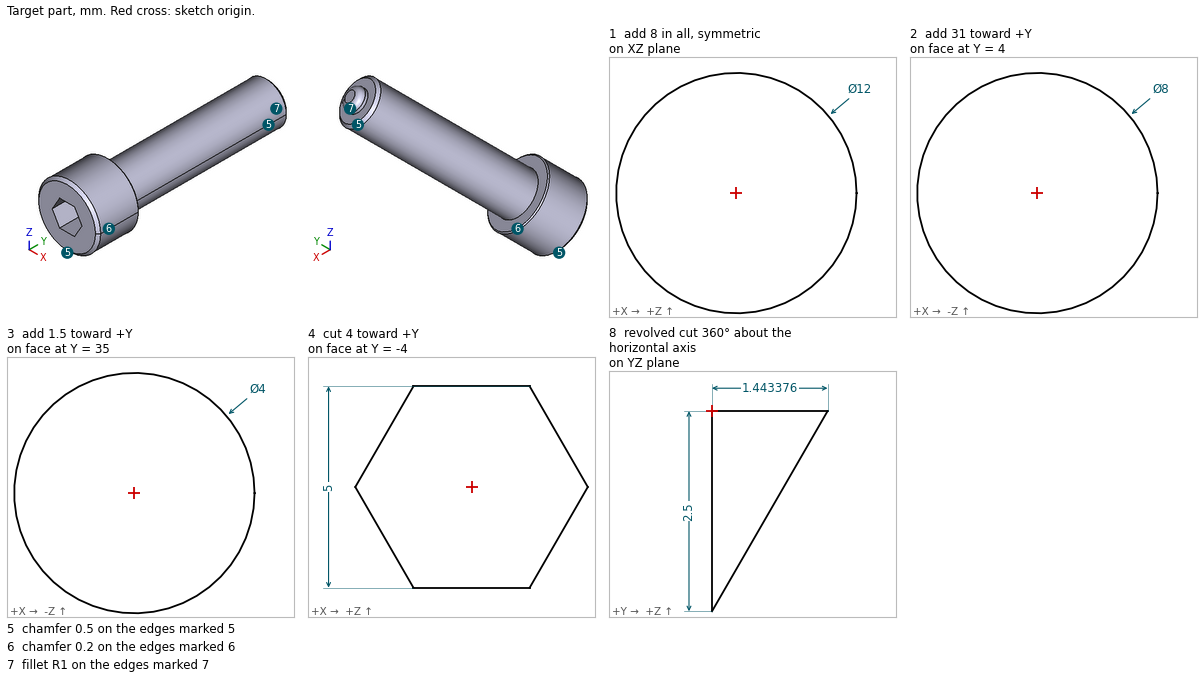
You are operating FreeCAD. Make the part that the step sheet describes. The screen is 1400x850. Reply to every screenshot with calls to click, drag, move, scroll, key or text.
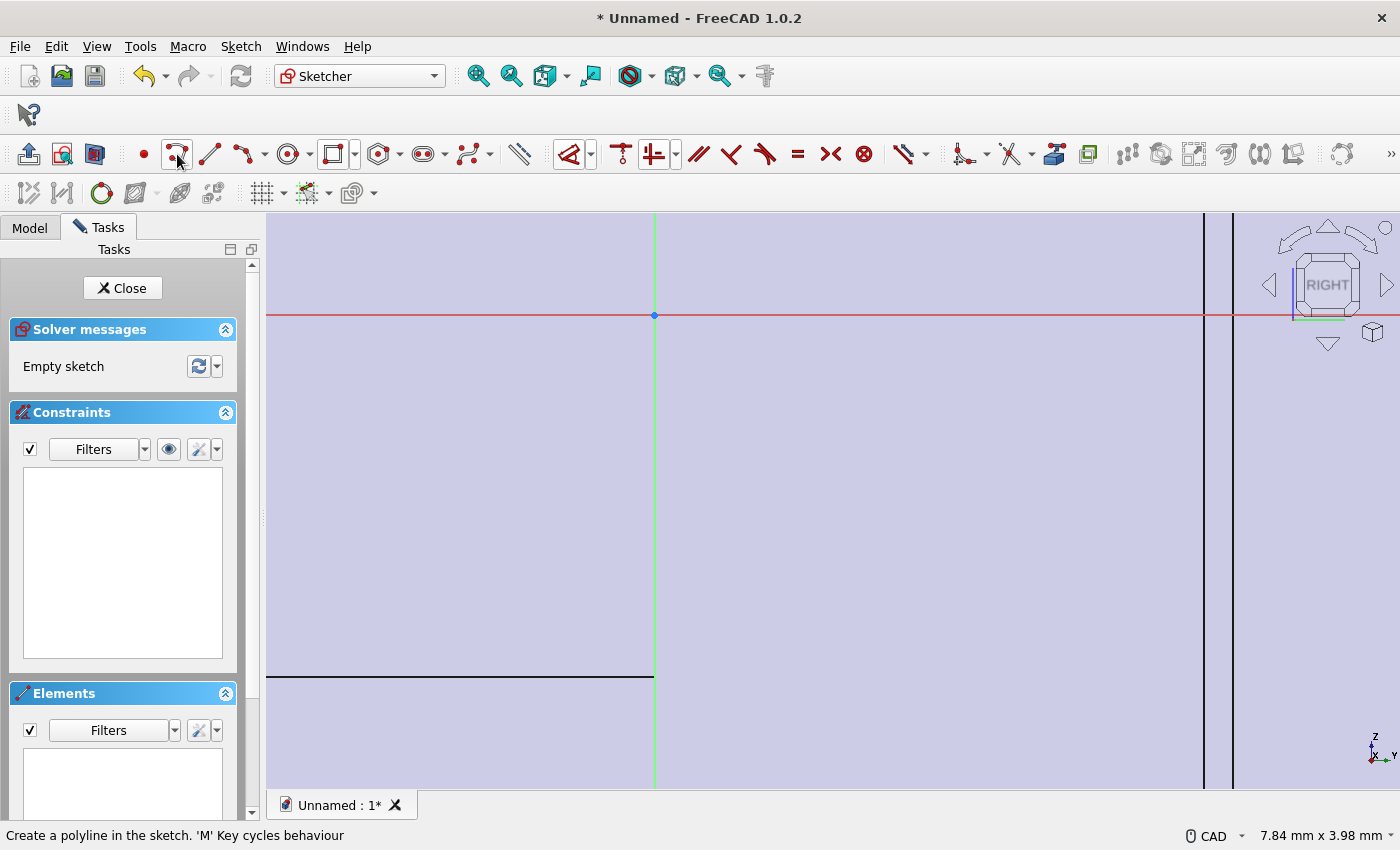
click(655, 315)
click(664, 677)
click(863, 324)
click(655, 315)
key(Escape)
key(Escape)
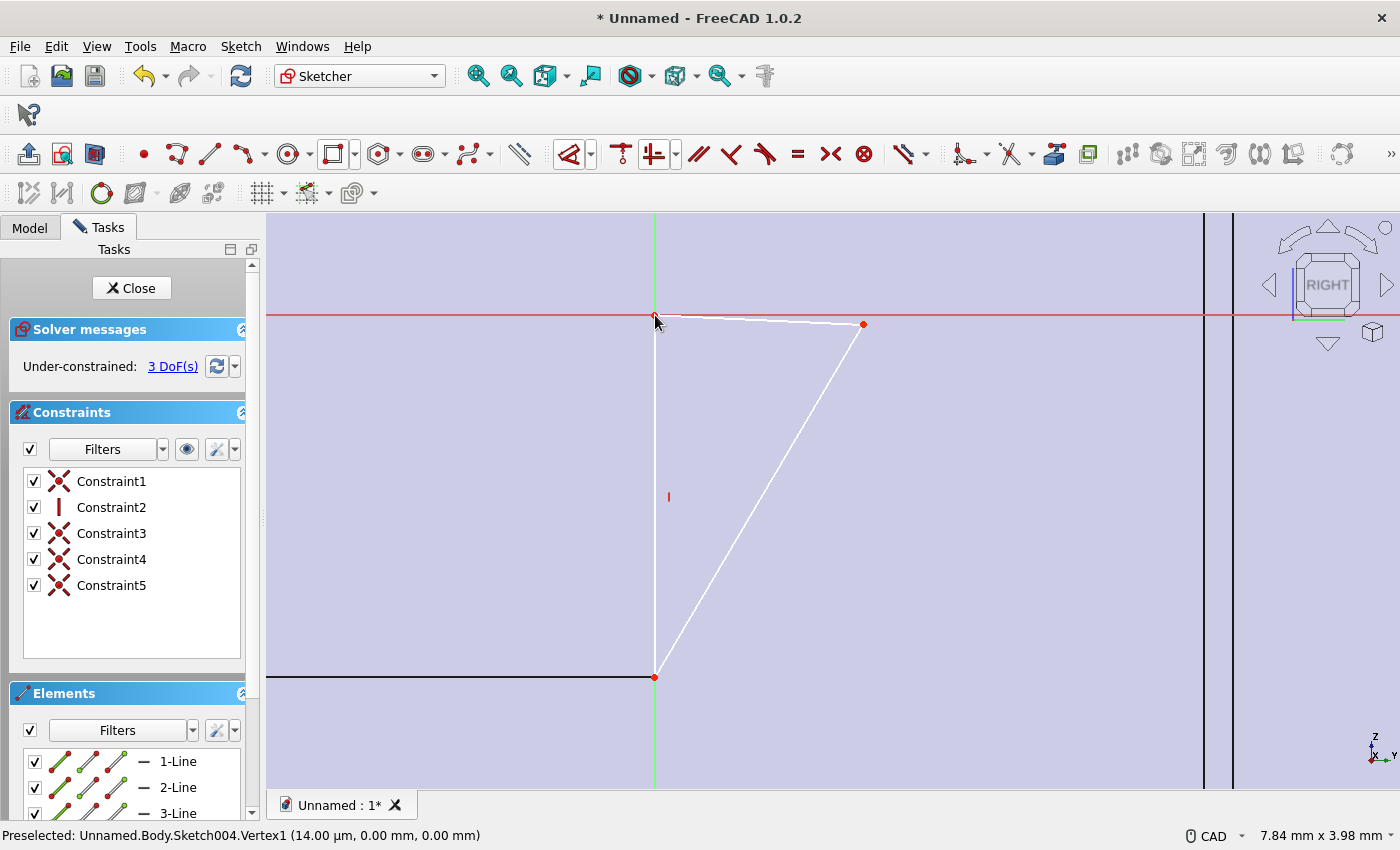
click(717, 318)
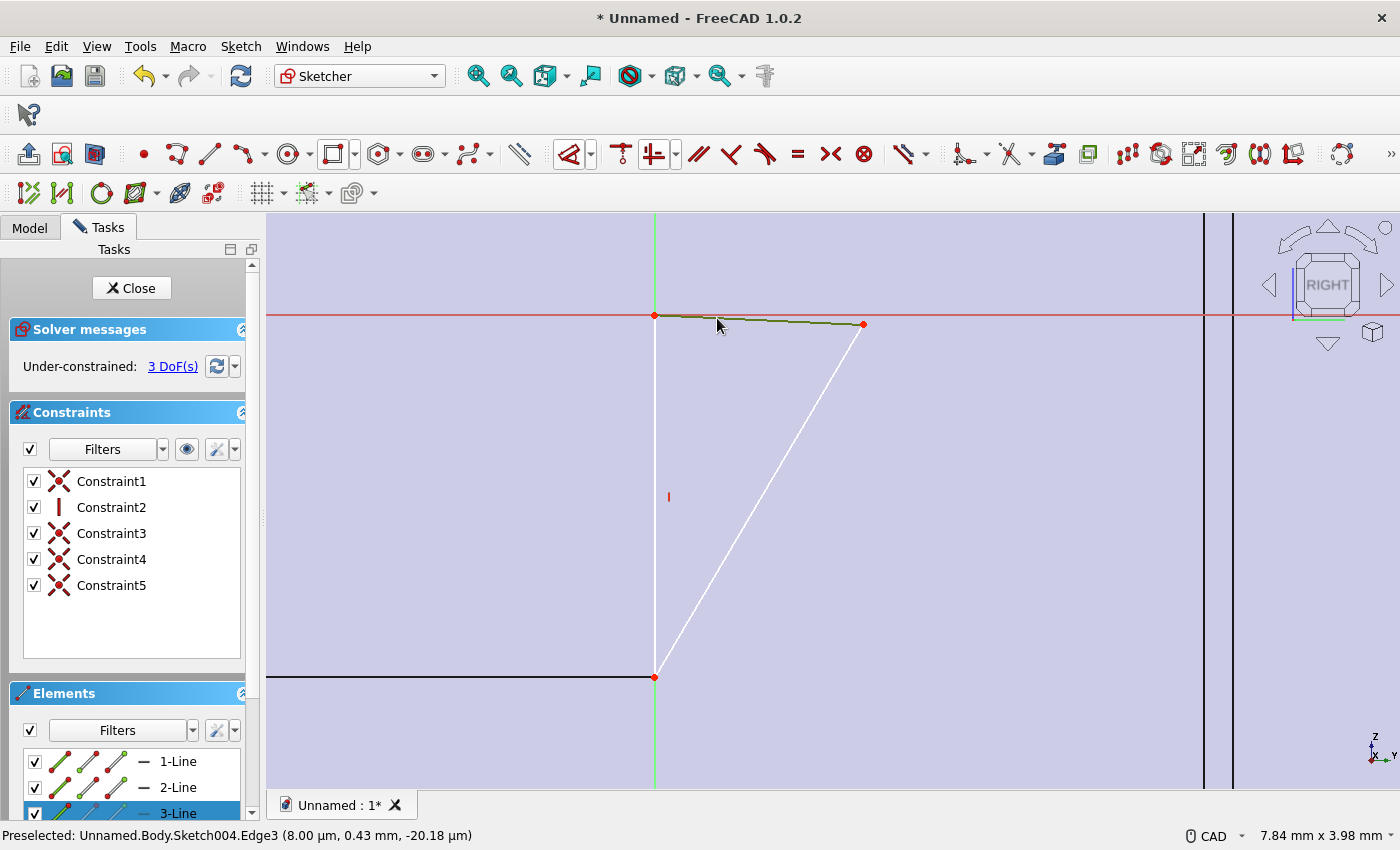
click(676, 154)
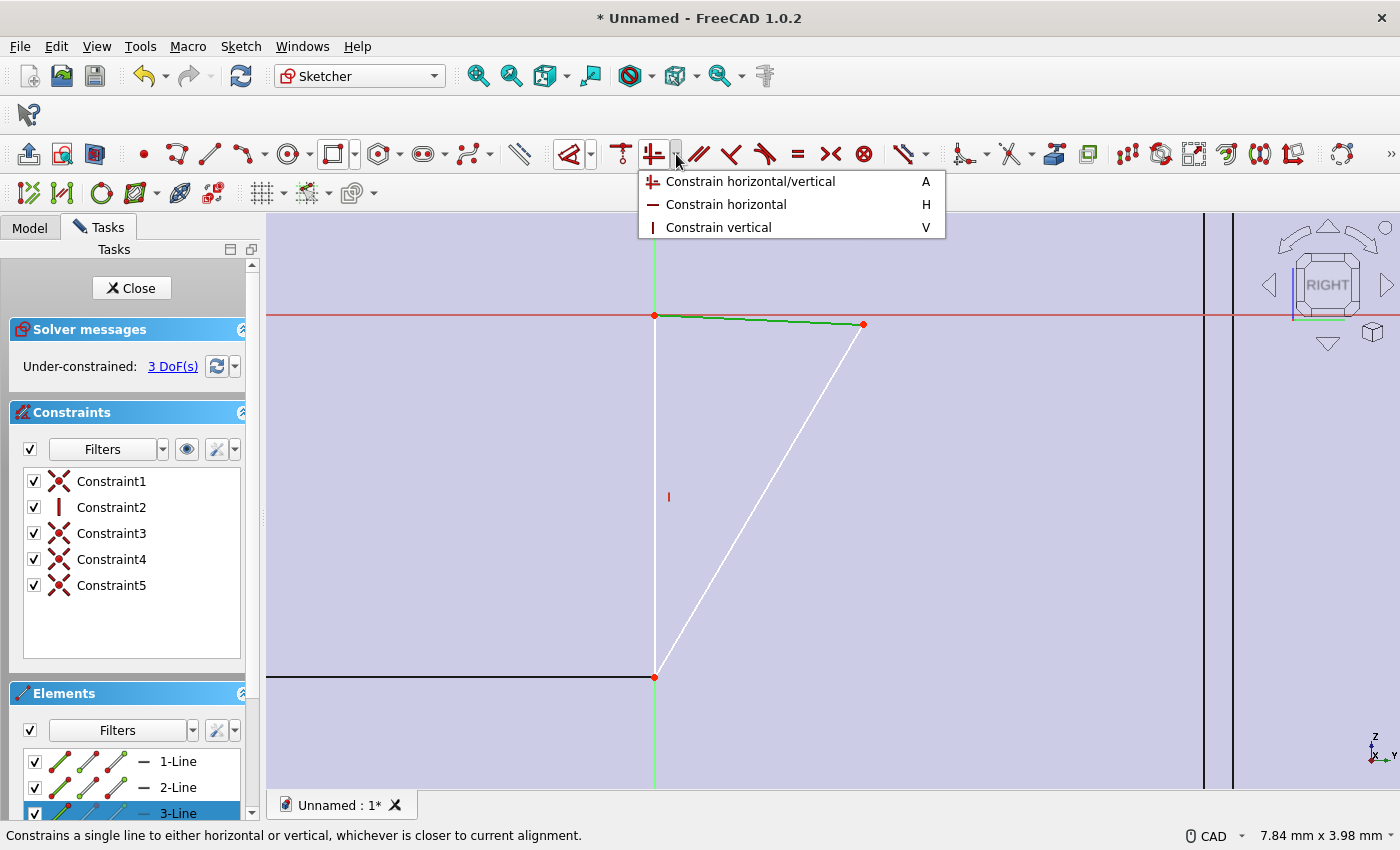
click(792, 204)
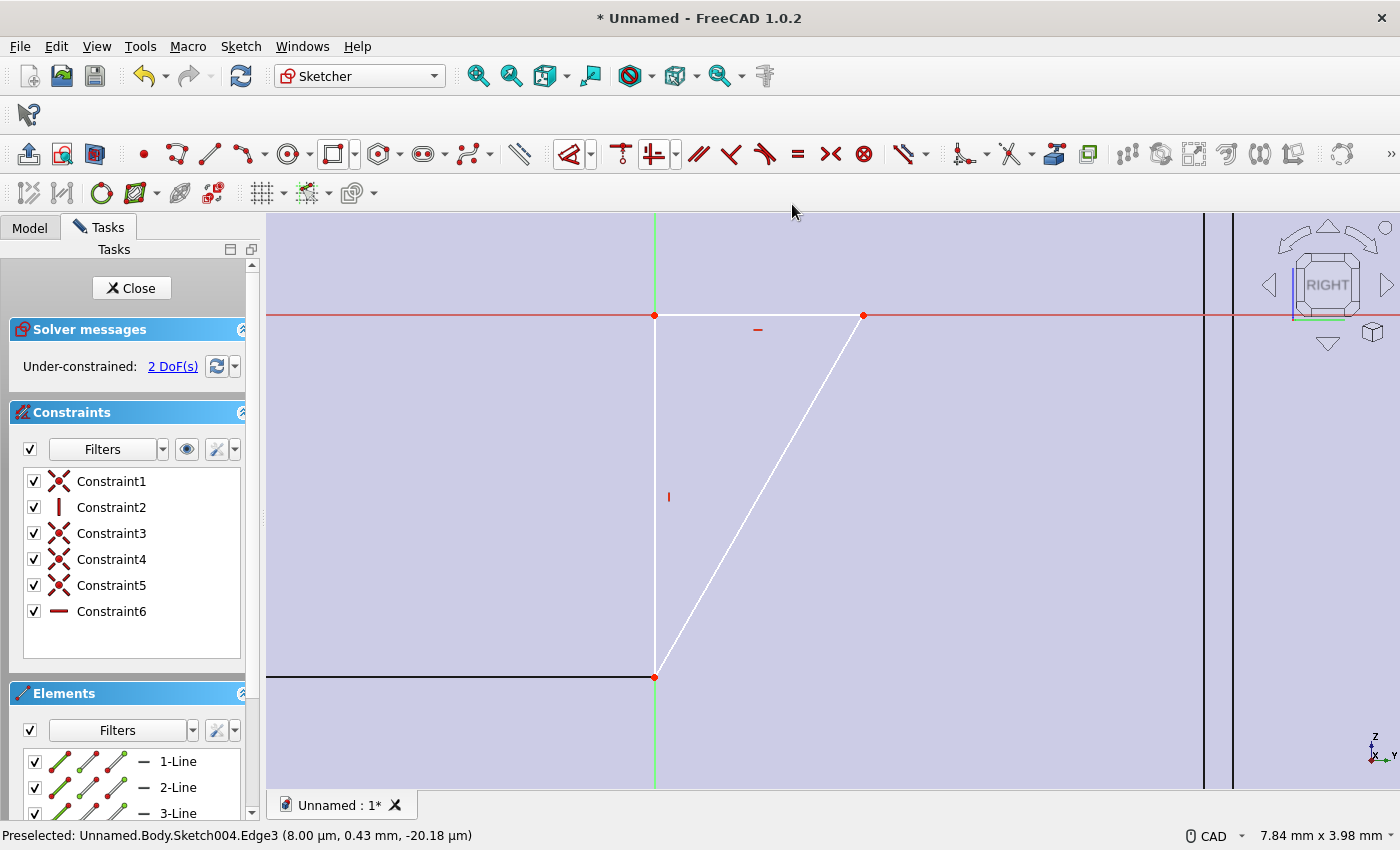
click(655, 424)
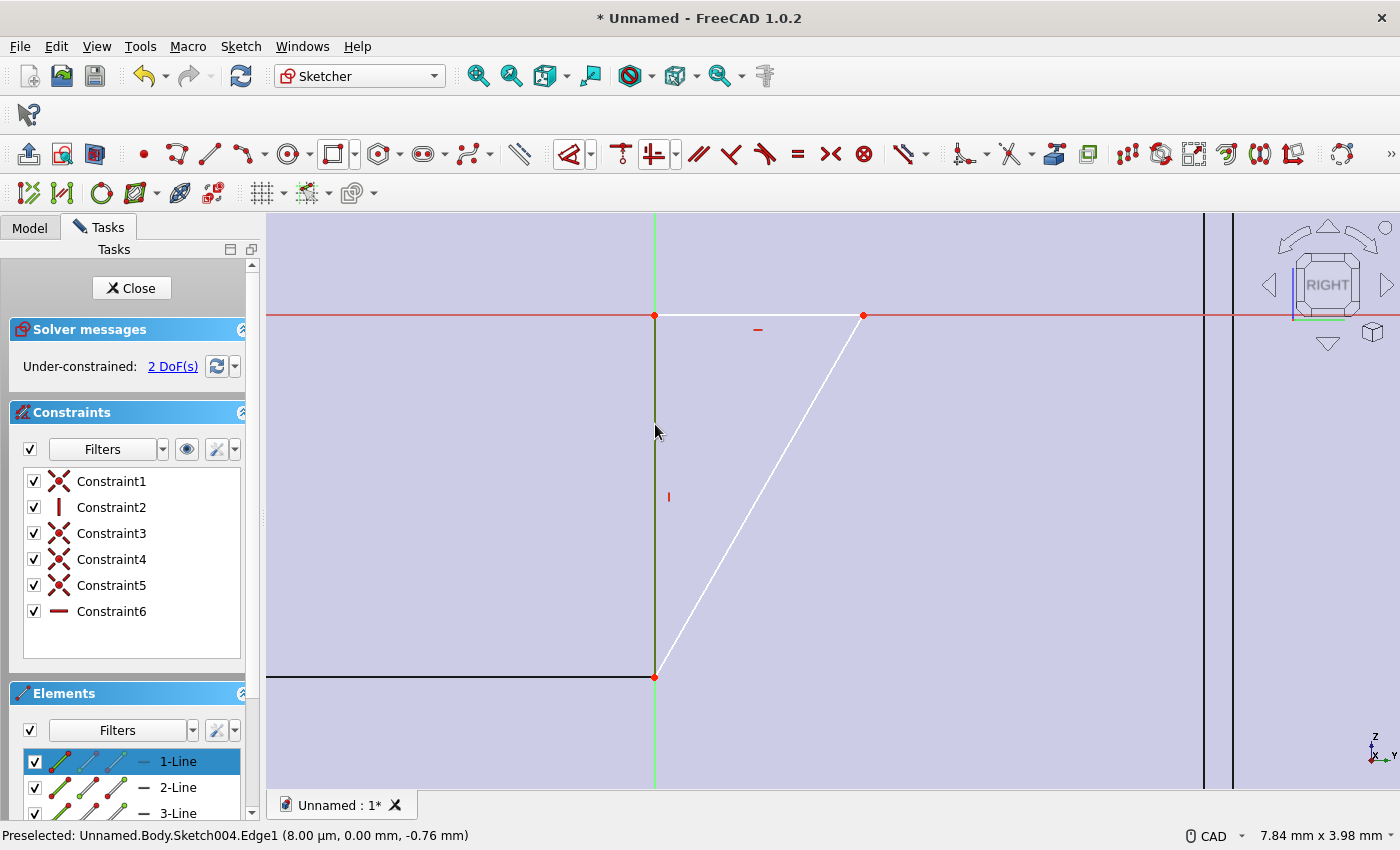
click(590, 154)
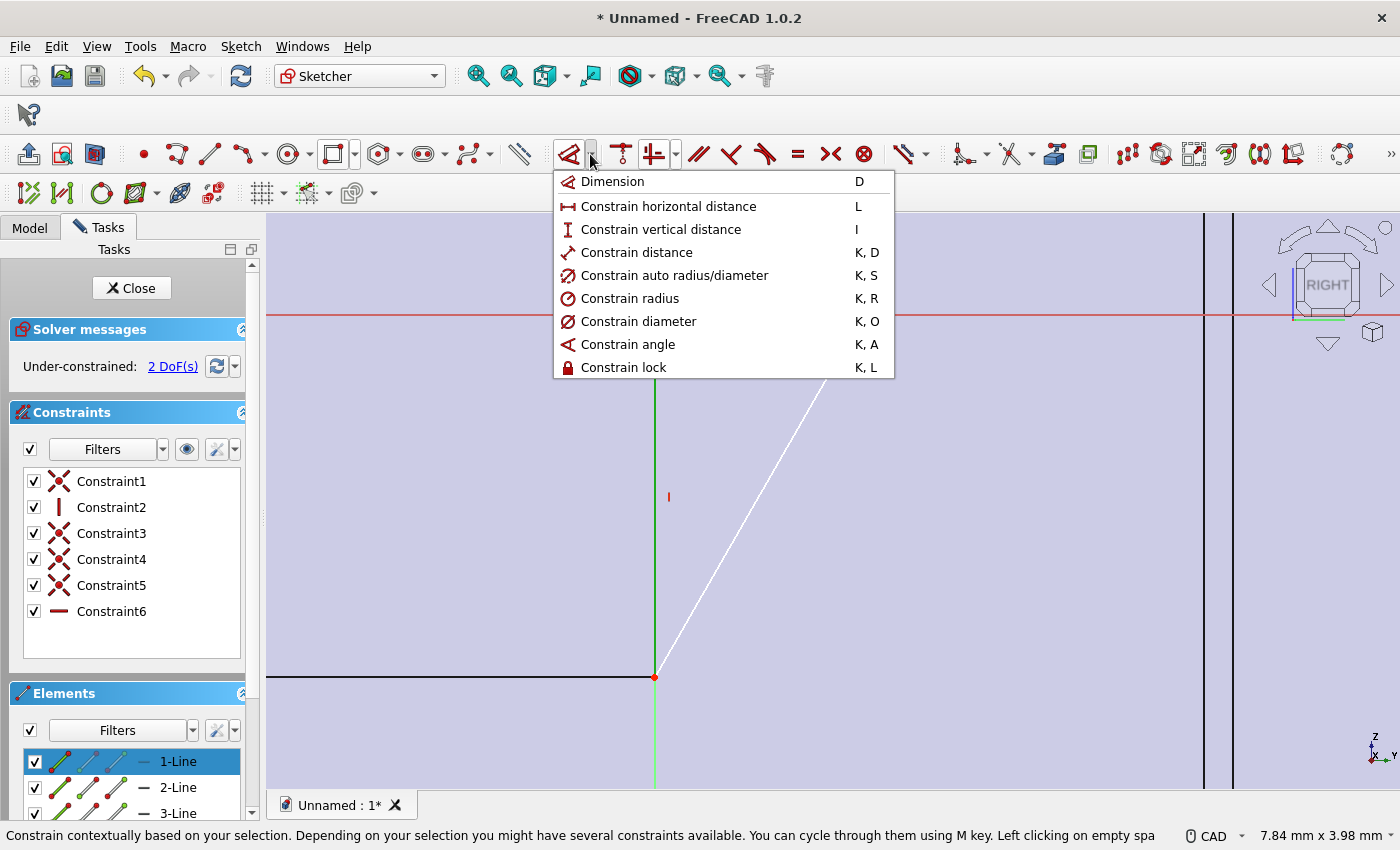
click(724, 230)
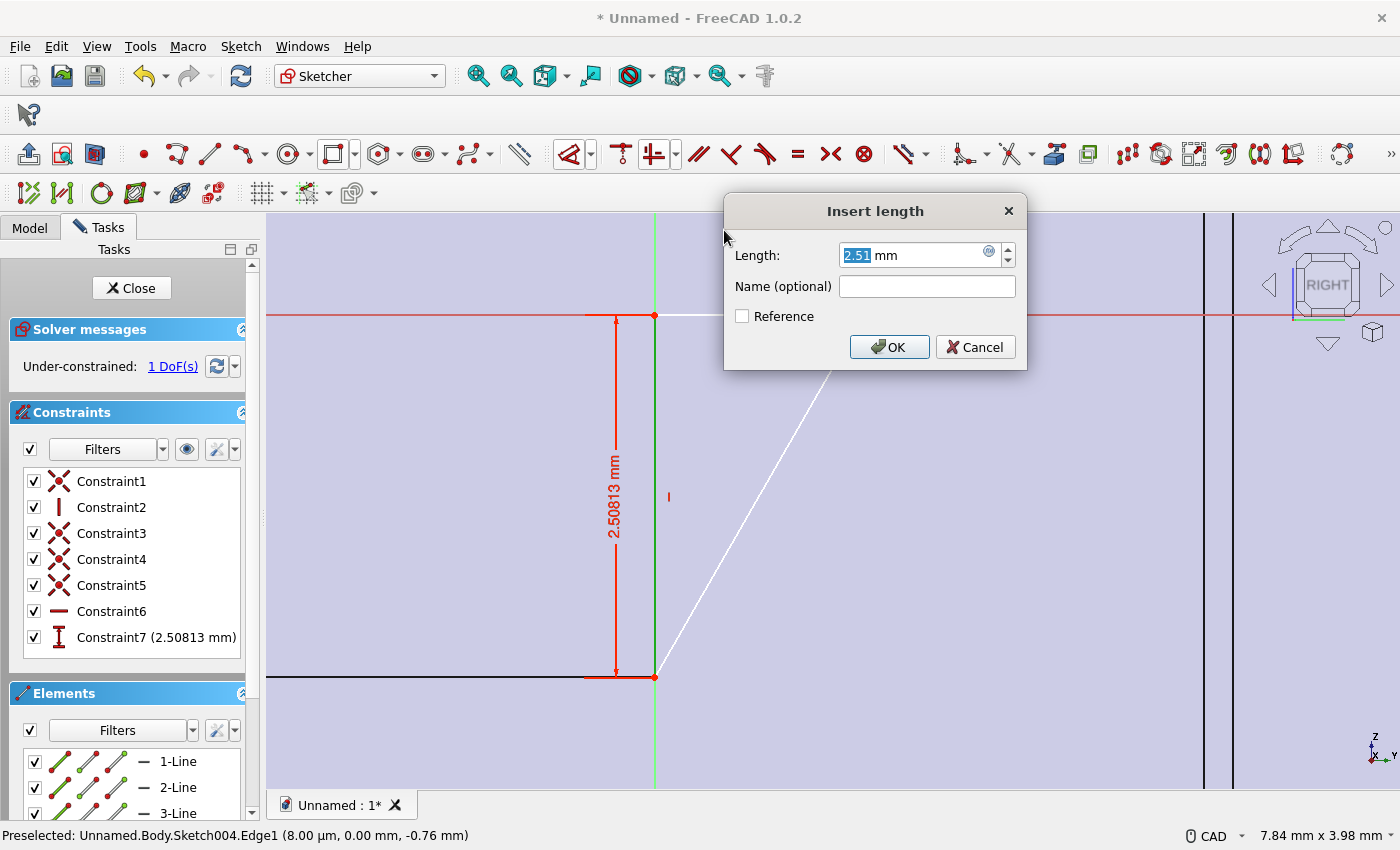
text(2.5)
key(Return)